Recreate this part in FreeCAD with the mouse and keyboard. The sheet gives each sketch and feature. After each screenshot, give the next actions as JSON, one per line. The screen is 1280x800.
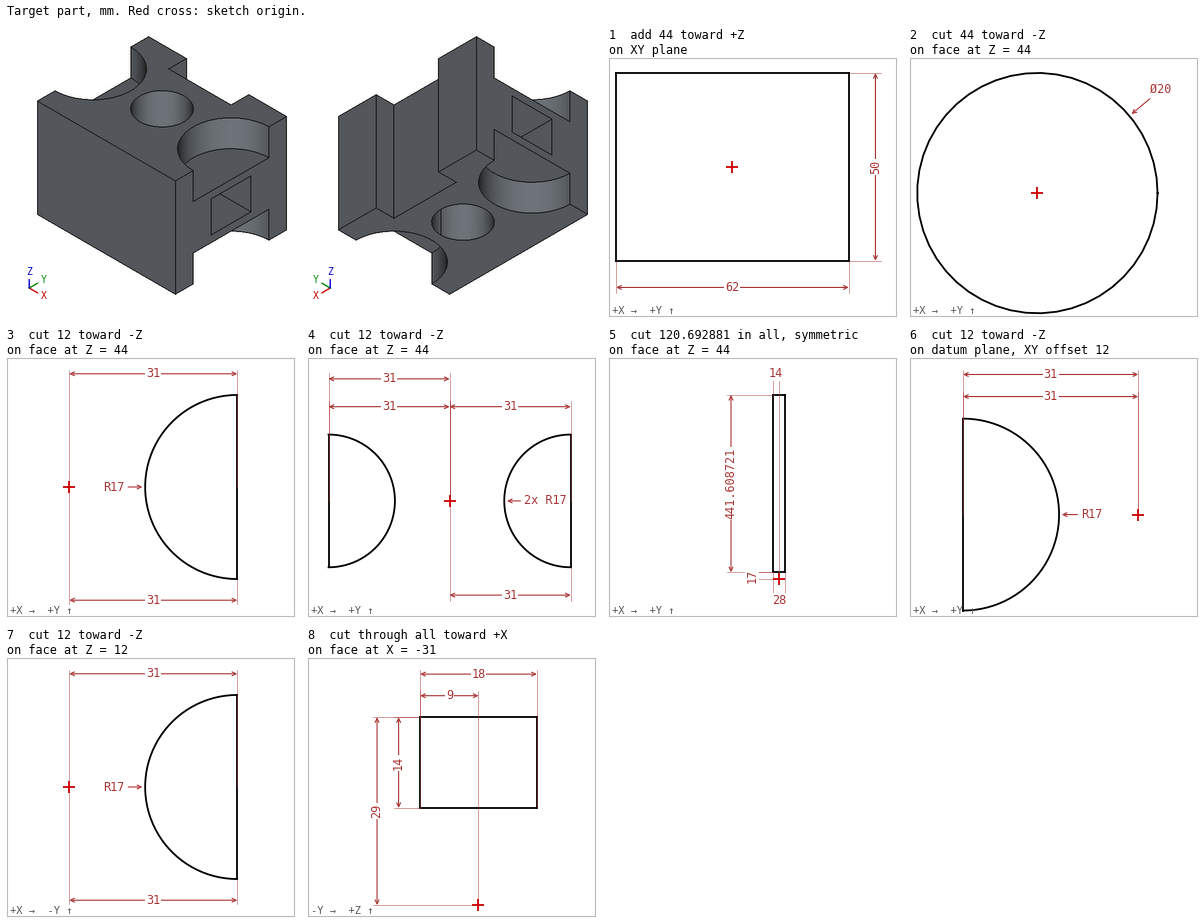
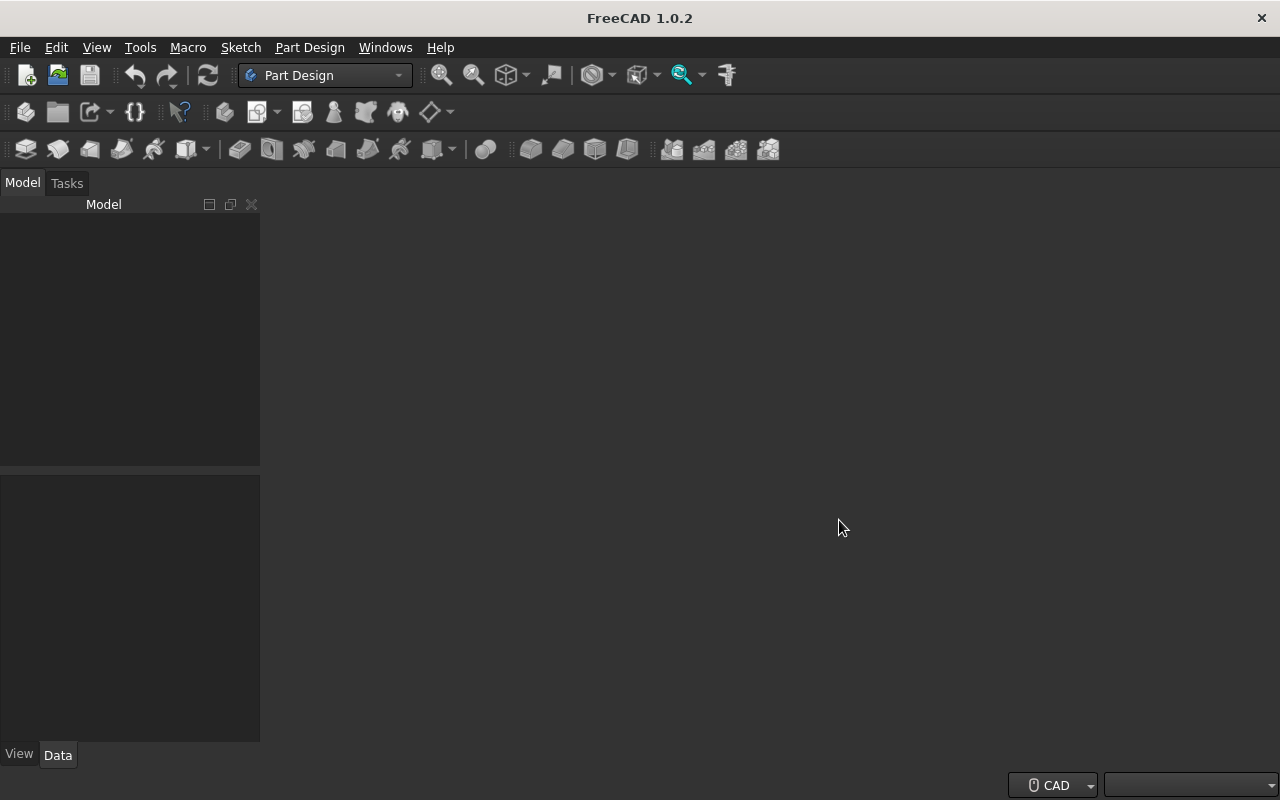
{"action": "key", "text": "ctrl+n"}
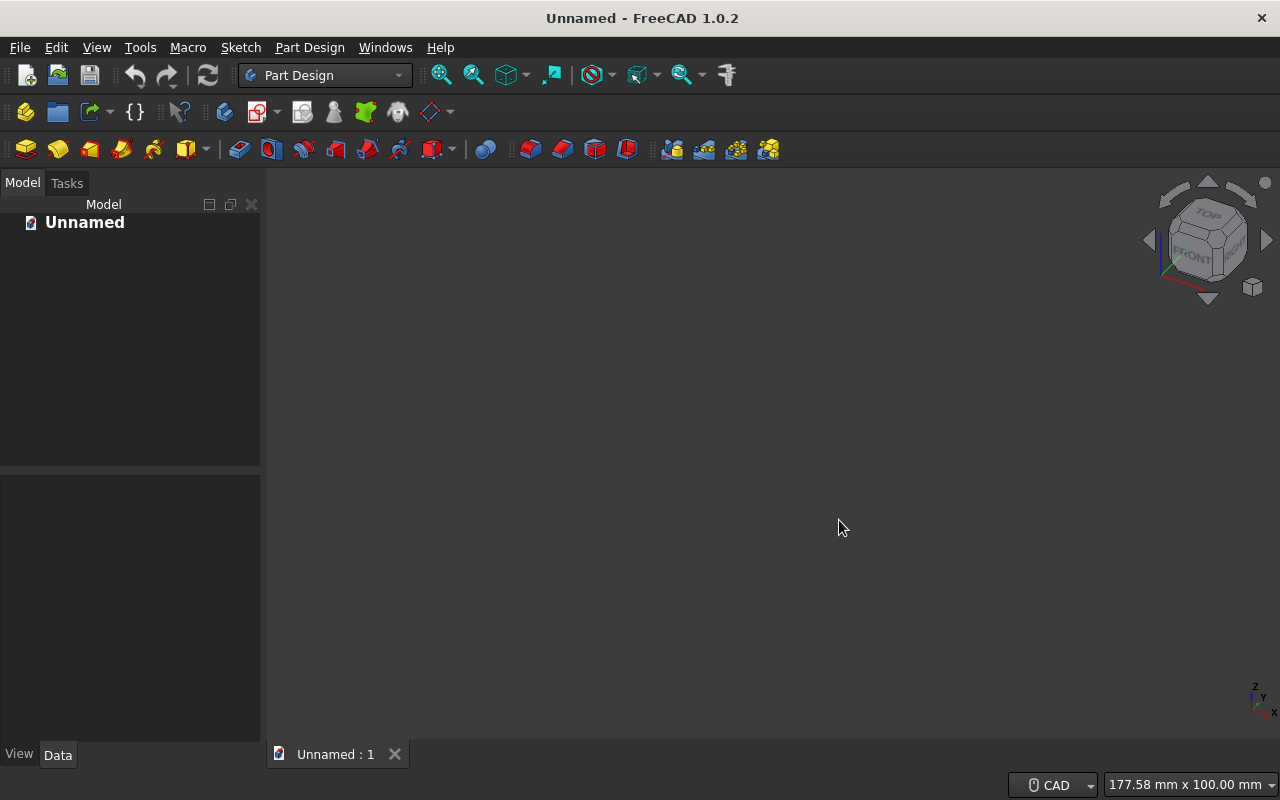
{"action": "left_click", "coordinate": [258, 112]}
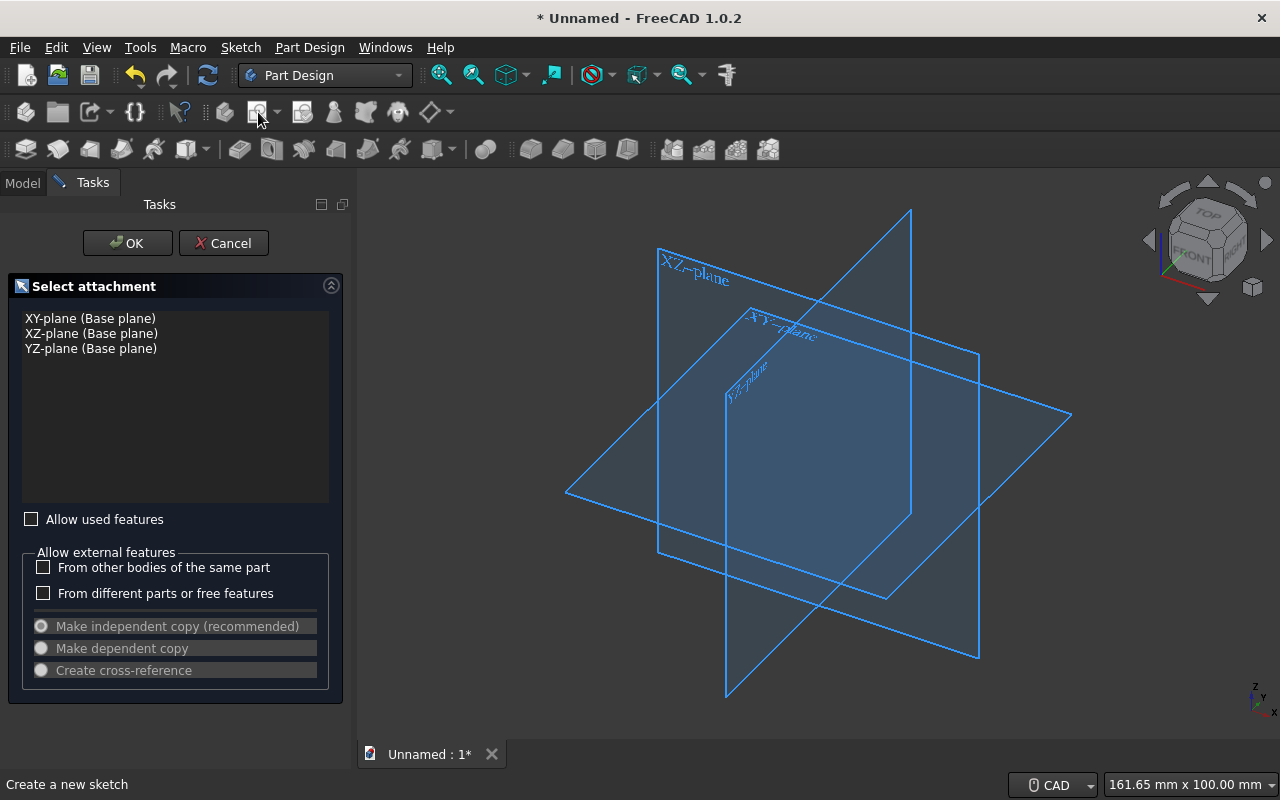
{"action": "left_click", "coordinate": [82, 318]}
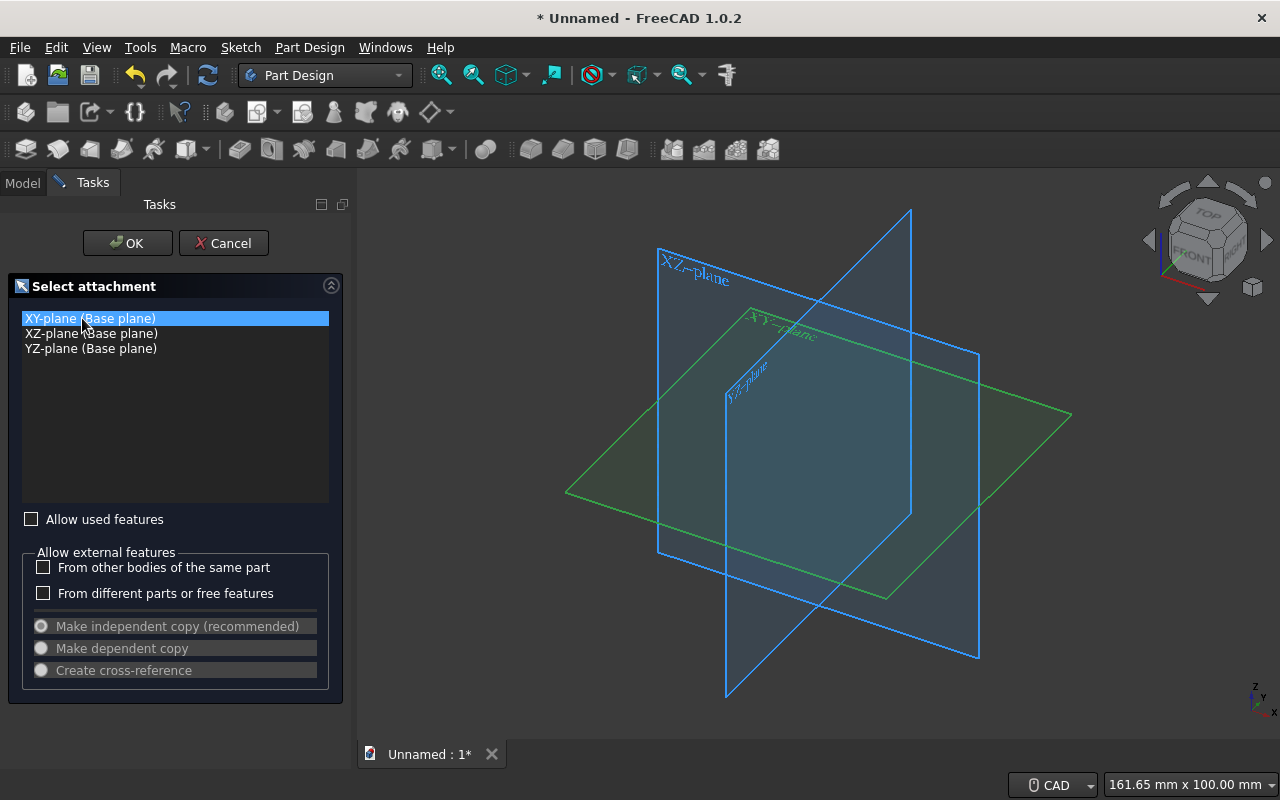
{"action": "left_click", "coordinate": [128, 243]}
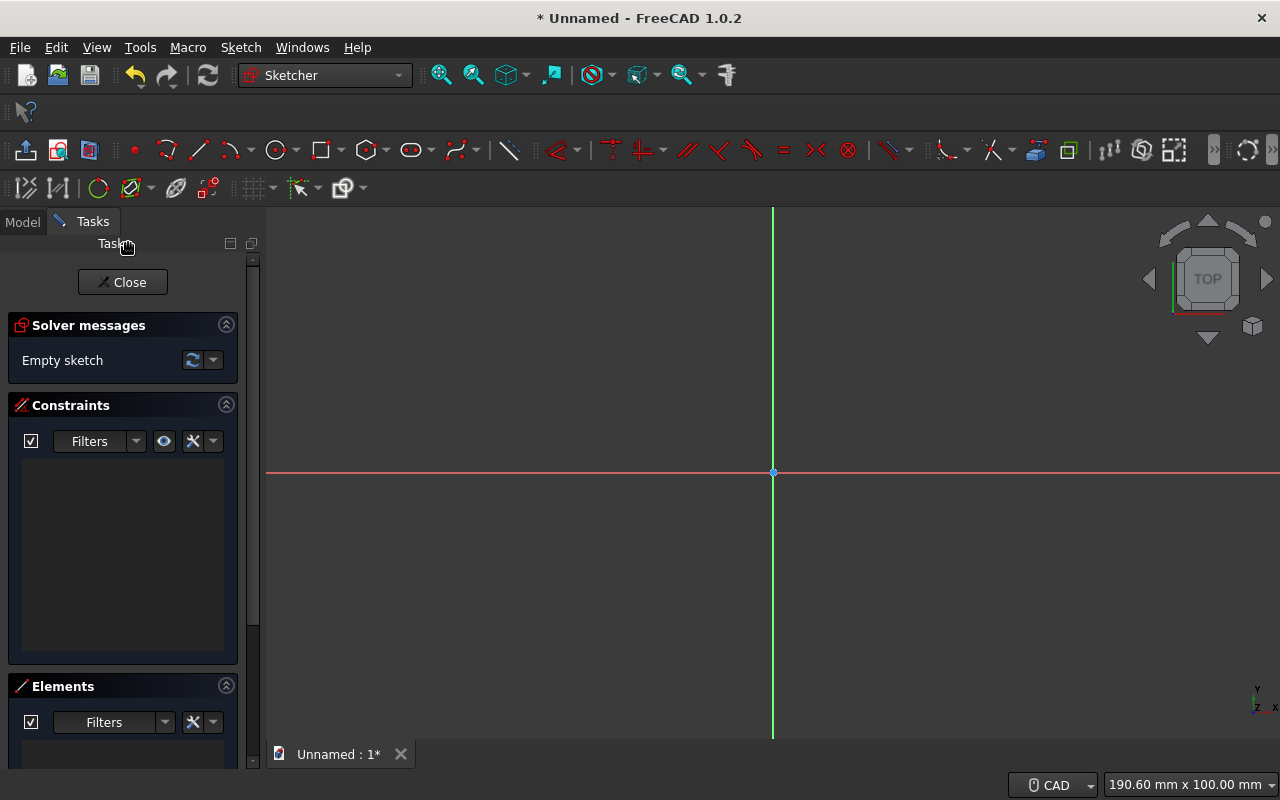
{"action": "key", "text": "g v"}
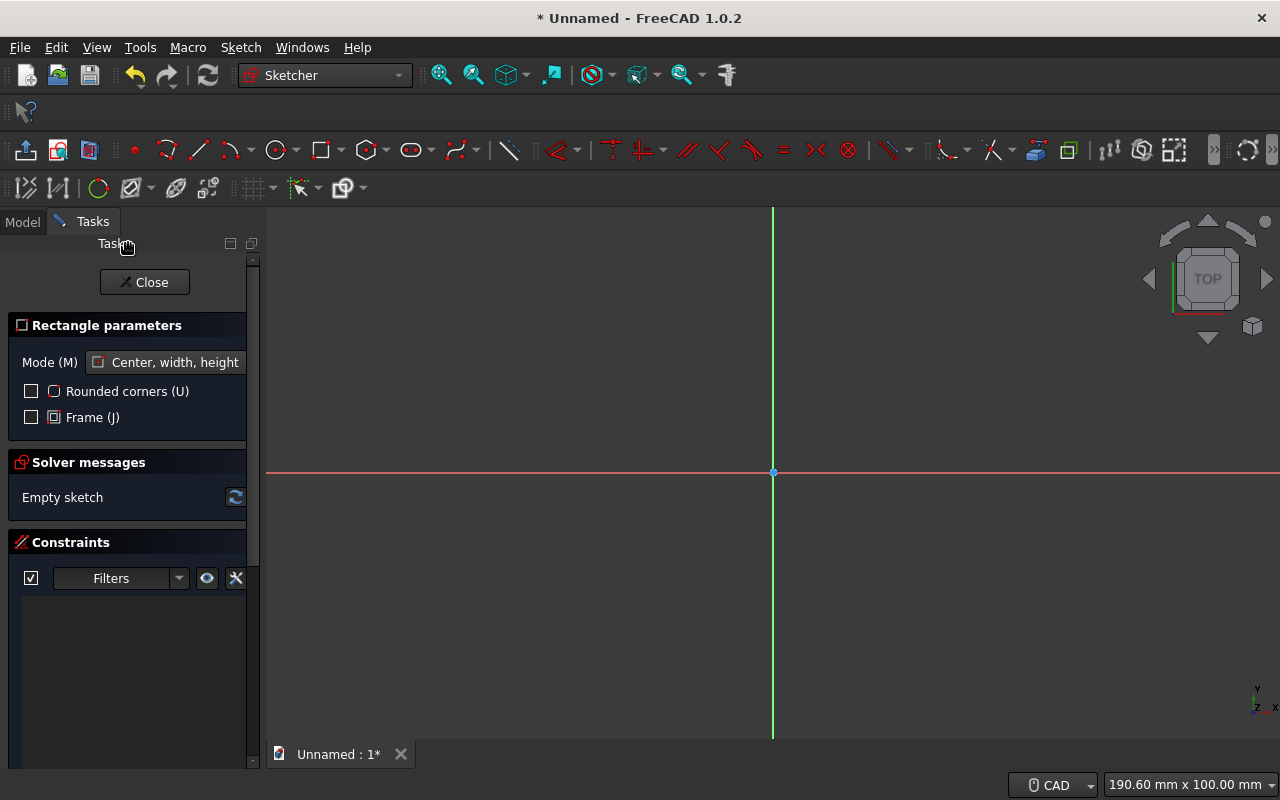
{"action": "left_click", "coordinate": [773, 473]}
{"action": "left_click", "coordinate": [938, 340]}
{"action": "key", "text": "Escape"}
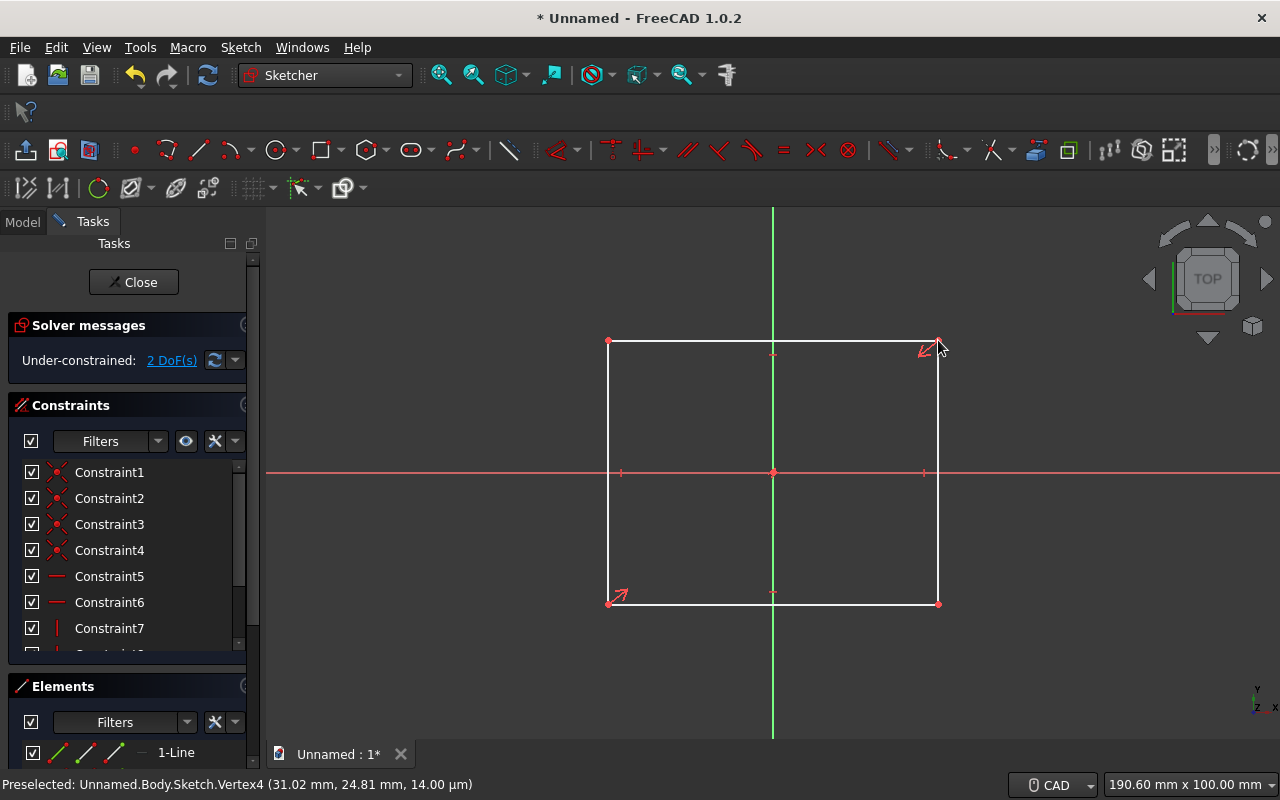
{"action": "left_click", "coordinate": [556, 150]}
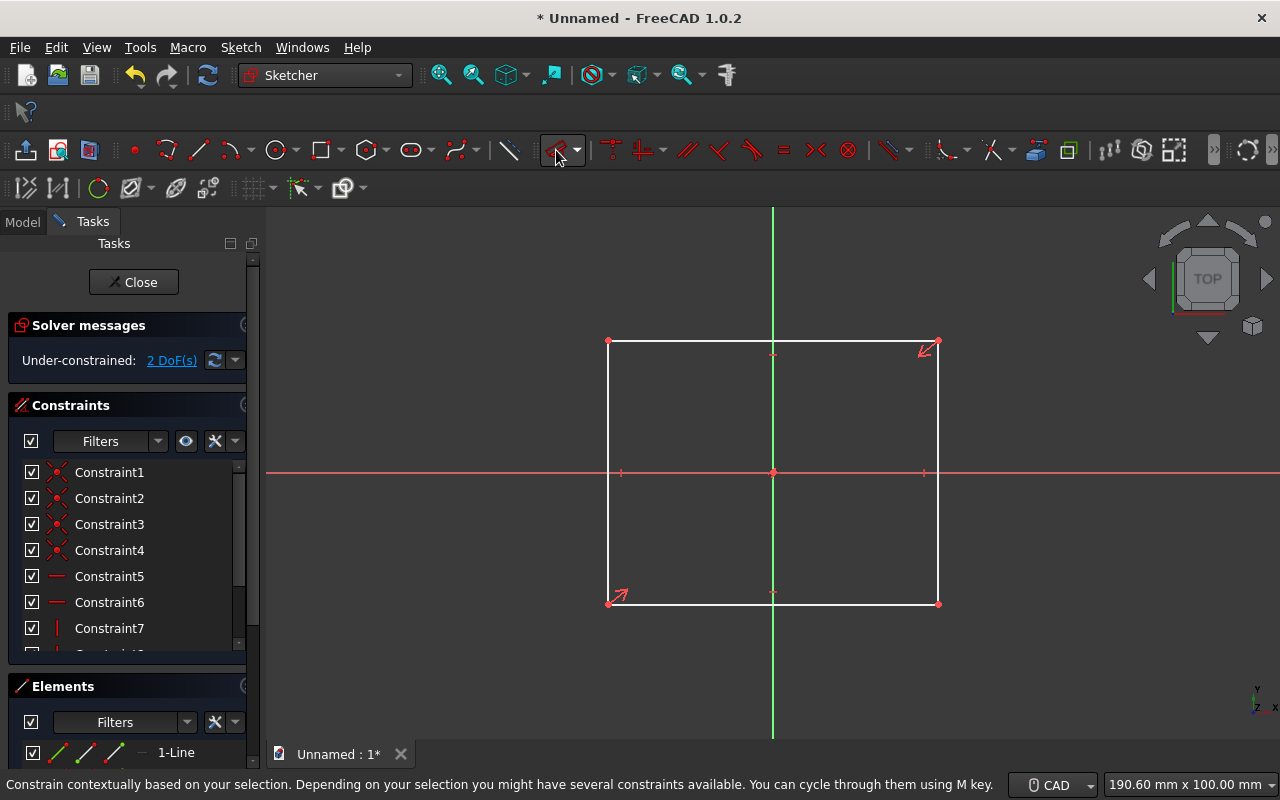
{"action": "left_click", "coordinate": [707, 605]}
{"action": "left_click", "coordinate": [697, 639]}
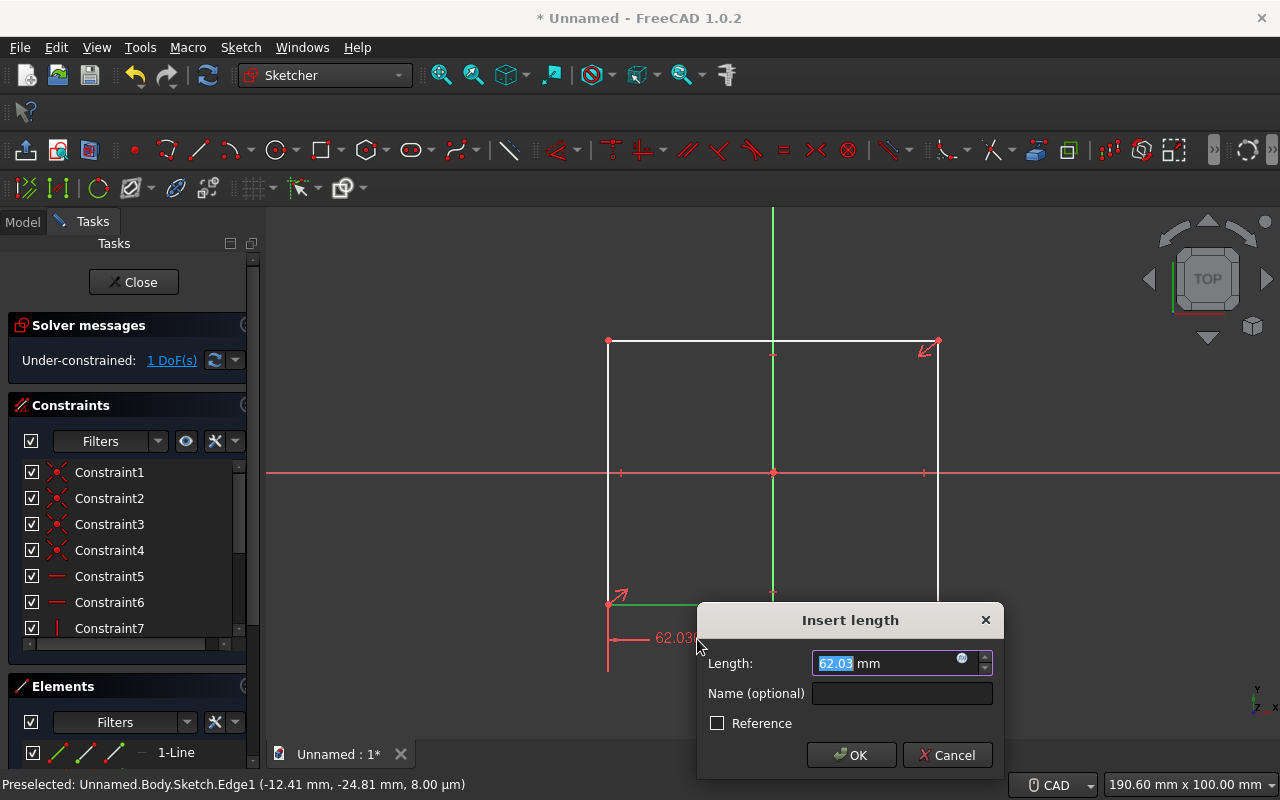
{"action": "type", "text": "62"}
{"action": "key", "text": "Return"}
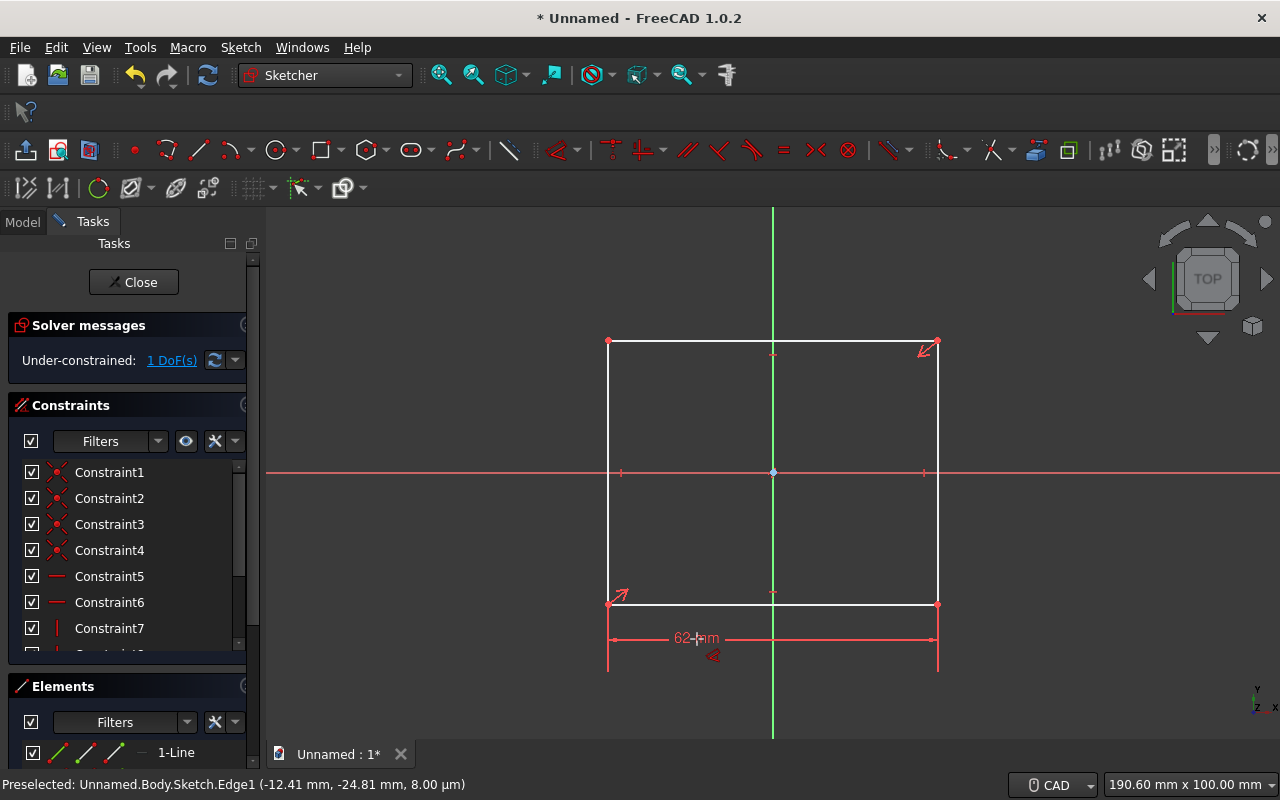
{"action": "left_click", "coordinate": [938, 526]}
{"action": "left_click", "coordinate": [972, 412]}